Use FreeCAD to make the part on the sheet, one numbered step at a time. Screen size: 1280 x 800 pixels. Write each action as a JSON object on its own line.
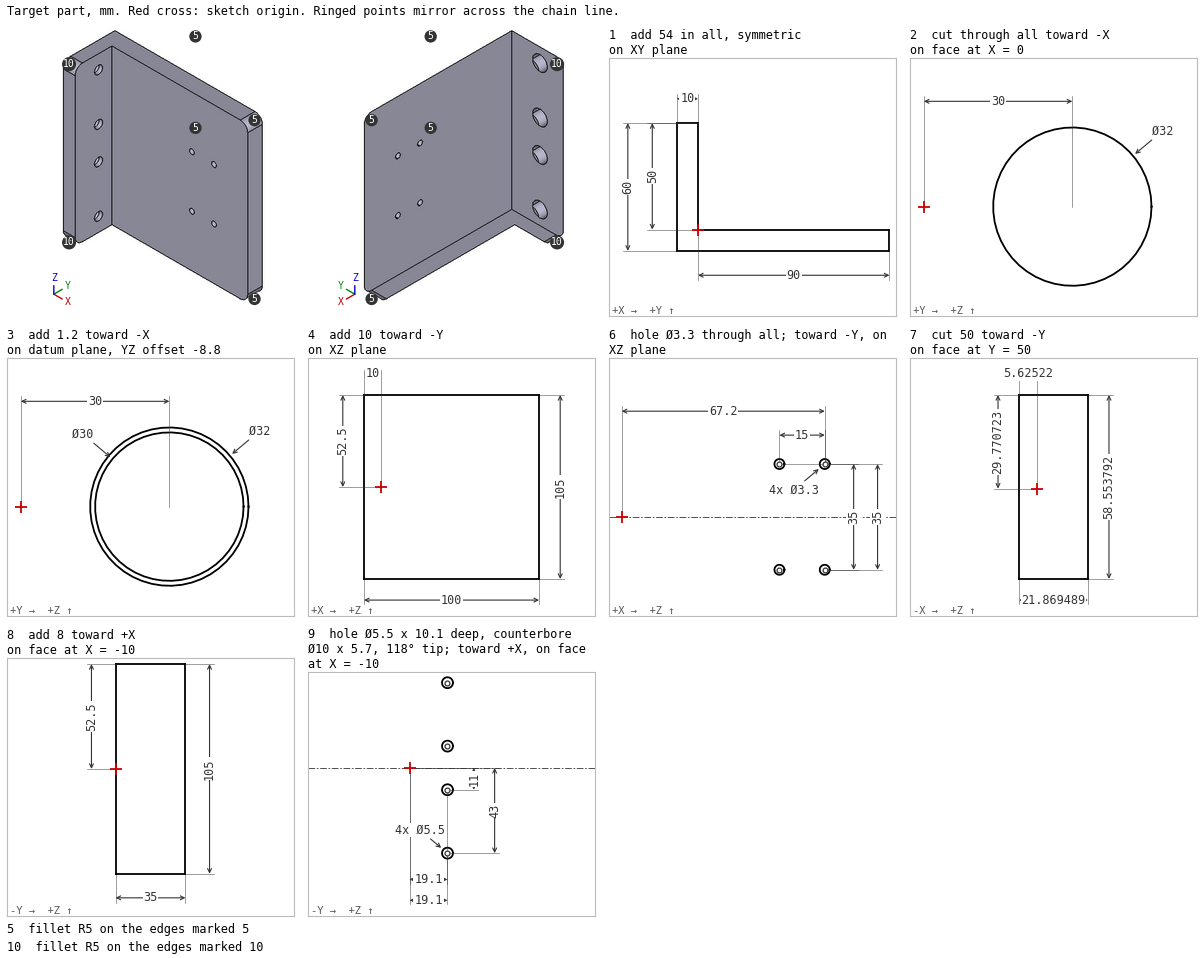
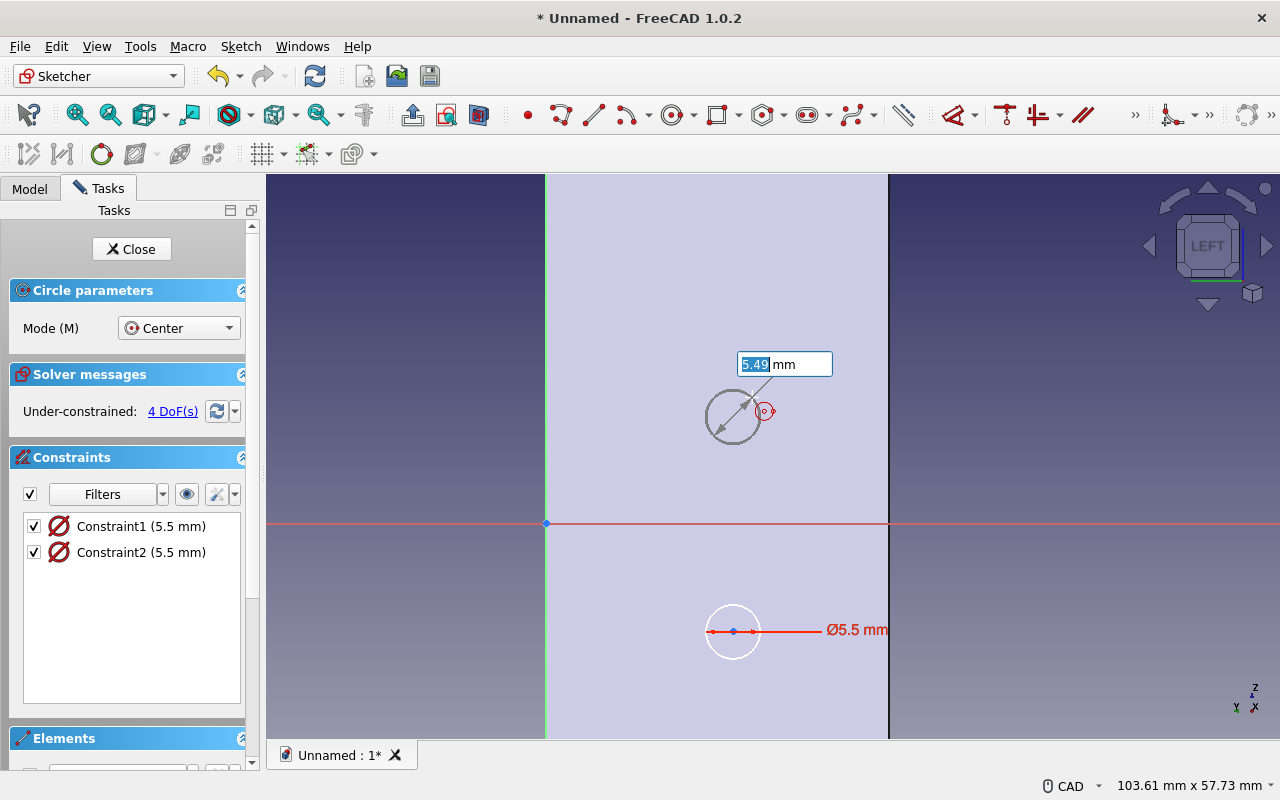
{"action": "type", "text": "5.5"}
{"action": "key", "text": "Return"}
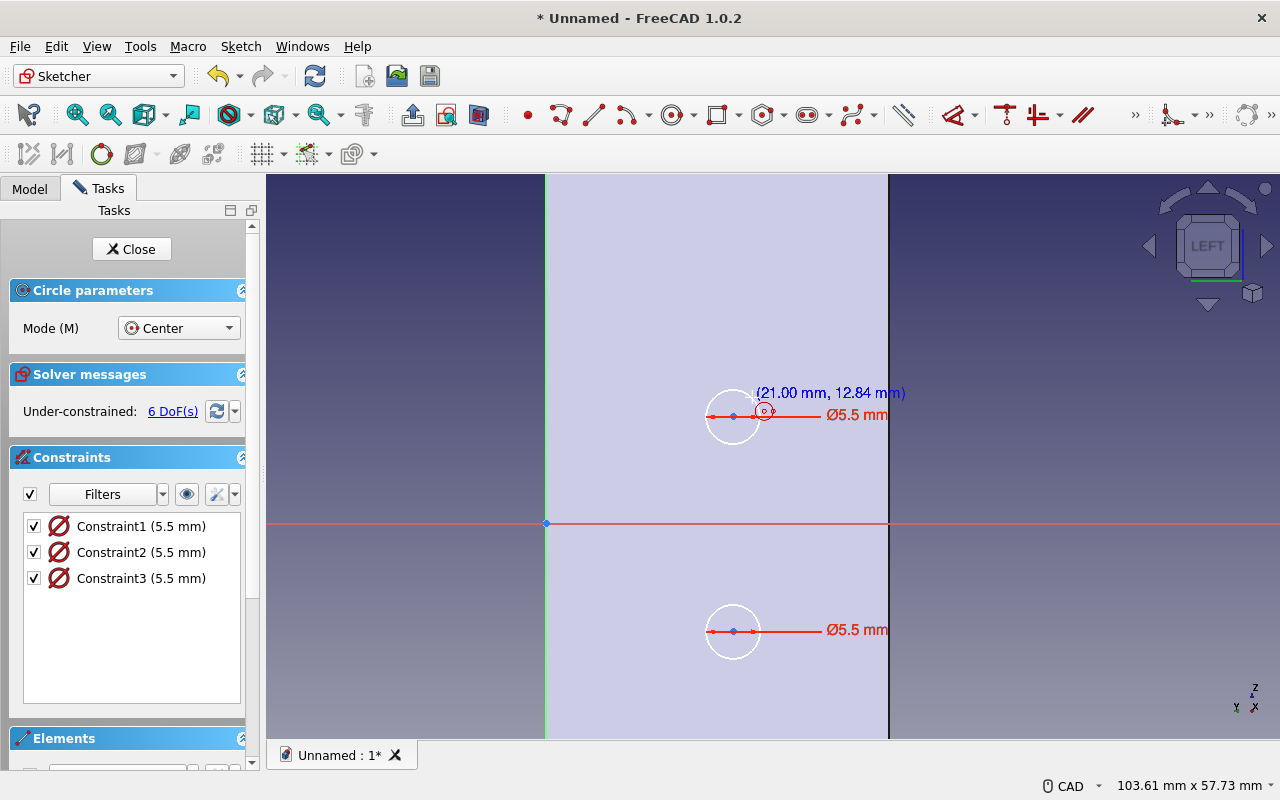
{"action": "scroll", "coordinate": [734, 417], "scroll_direction": "down", "scroll_amount": 5}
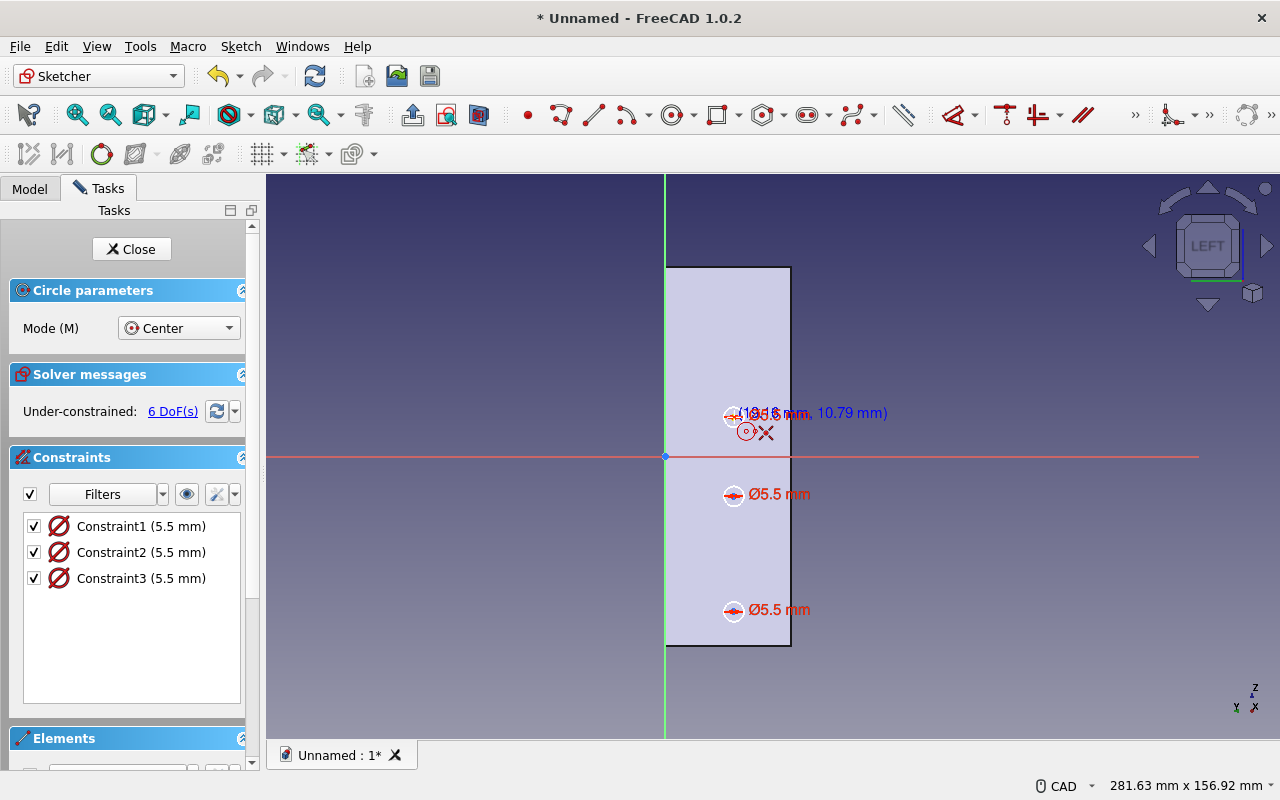
{"action": "scroll", "coordinate": [734, 302], "scroll_direction": "up", "scroll_amount": 5}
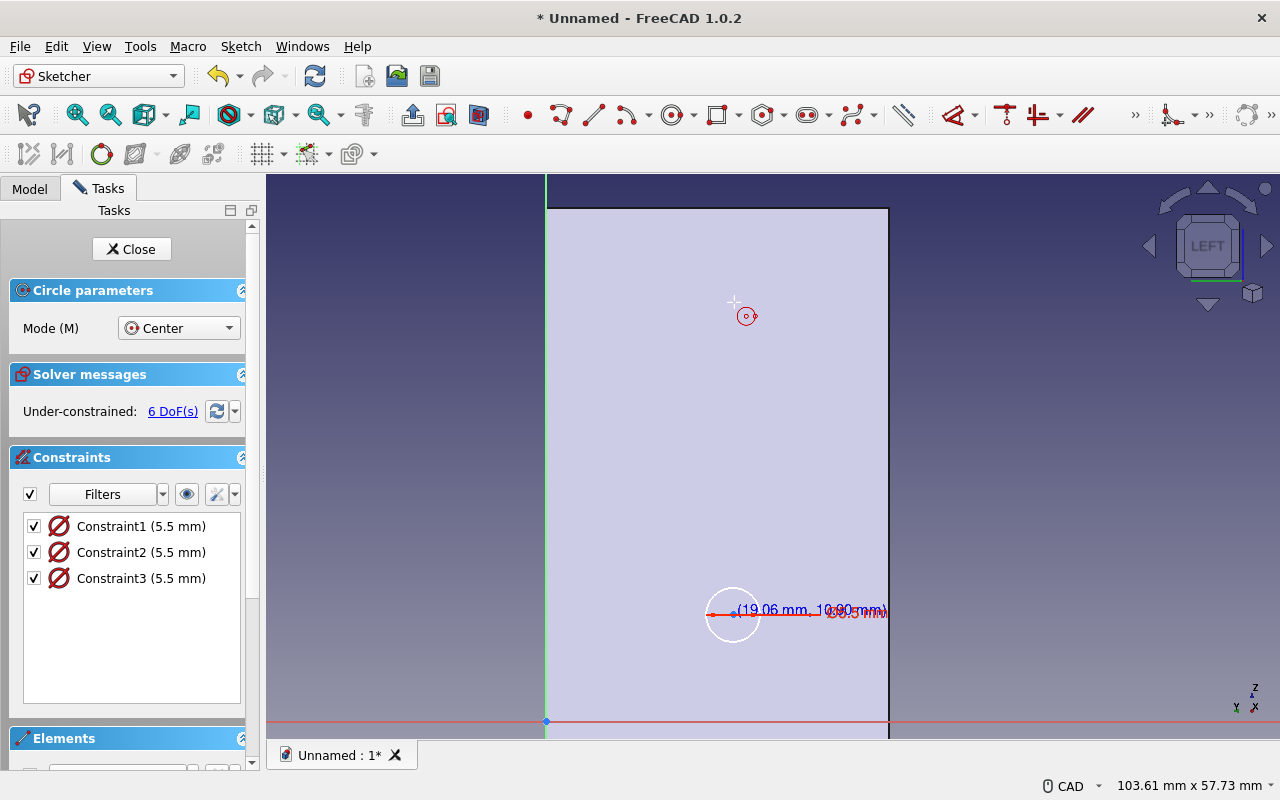
{"action": "left_click", "coordinate": [733, 301]}
{"action": "mouse_move", "coordinate": [752, 282]}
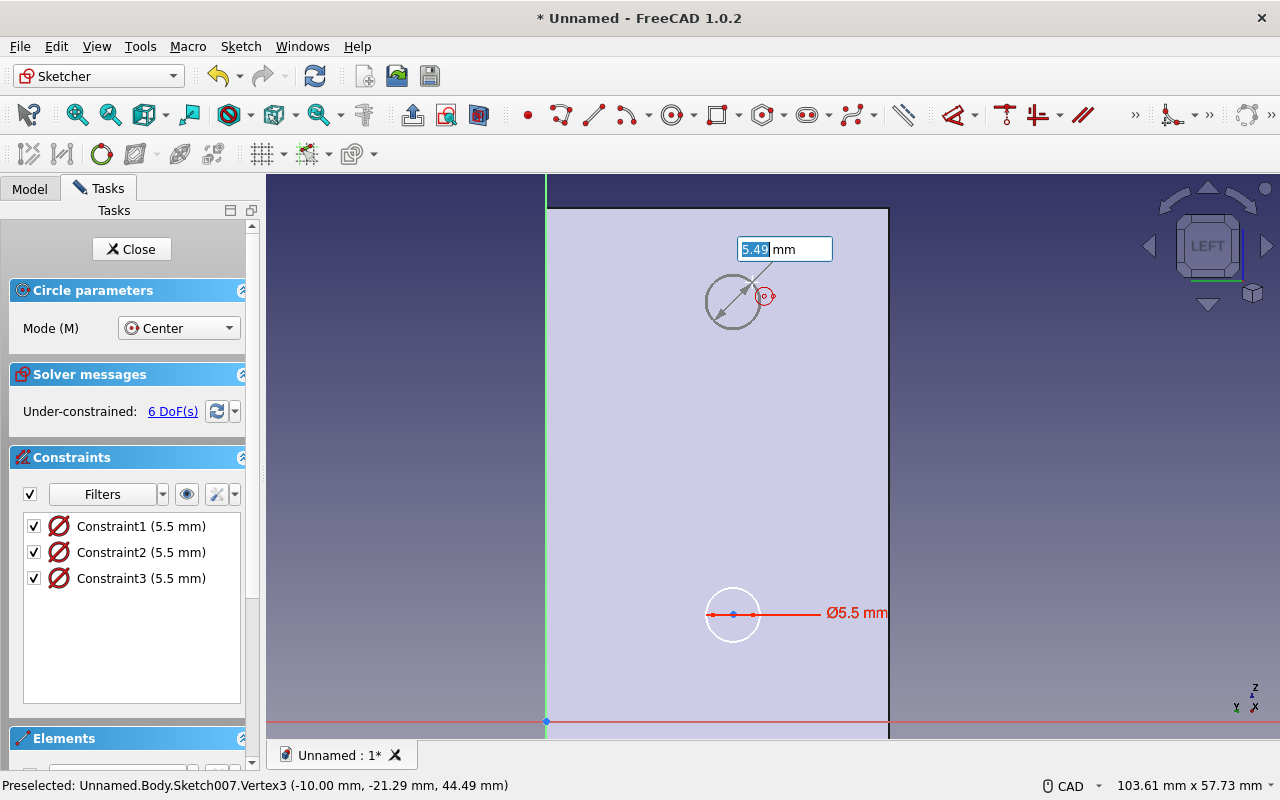
{"action": "type", "text": "5.5"}
{"action": "key", "text": "Return"}
{"action": "key", "text": "Escape"}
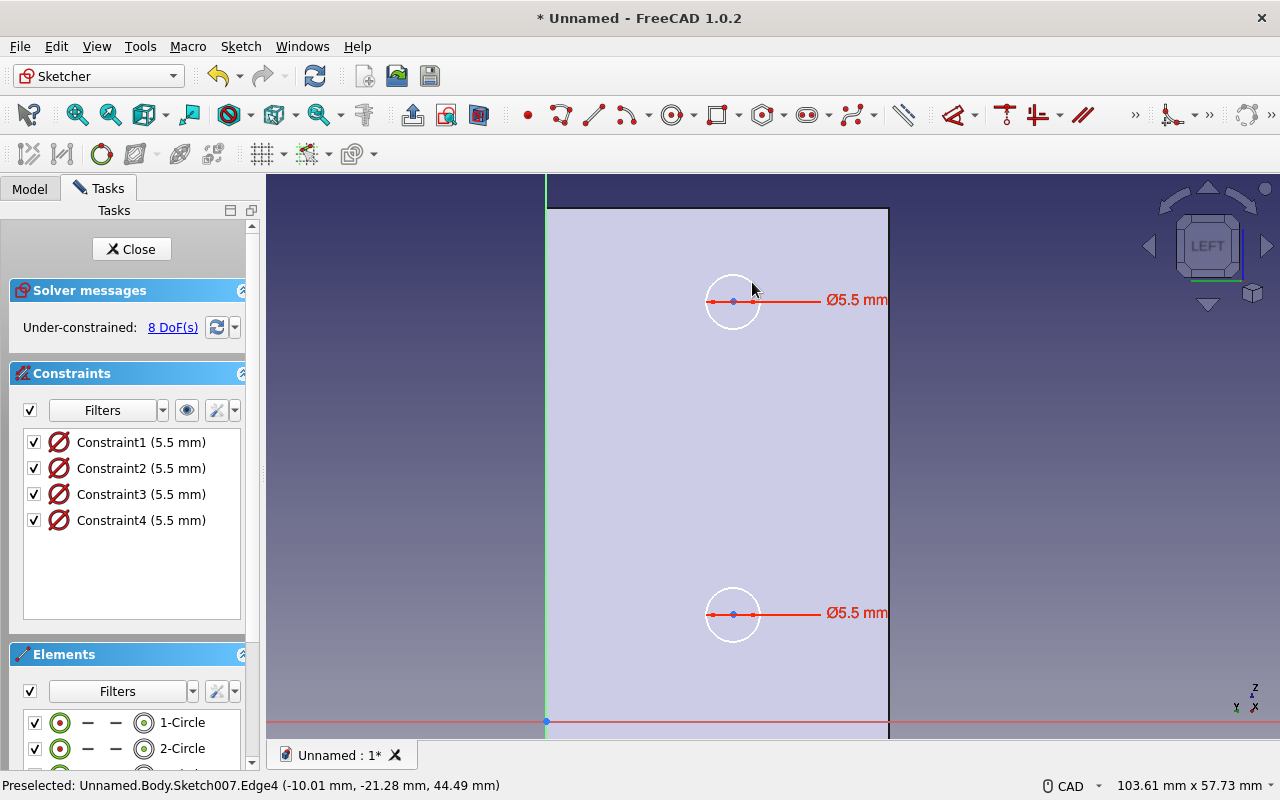
{"action": "scroll", "coordinate": [734, 302], "scroll_direction": "down", "scroll_amount": 5}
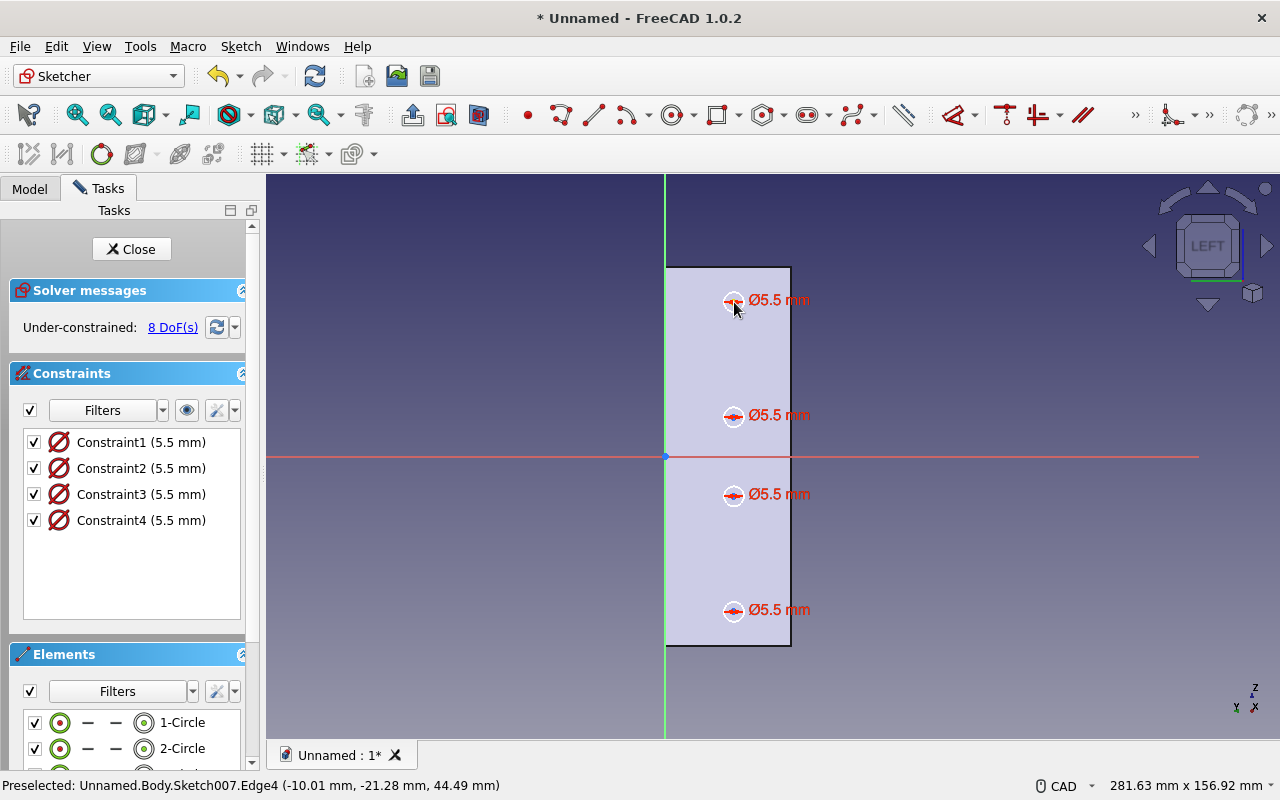
{"action": "left_click", "coordinate": [734, 496]}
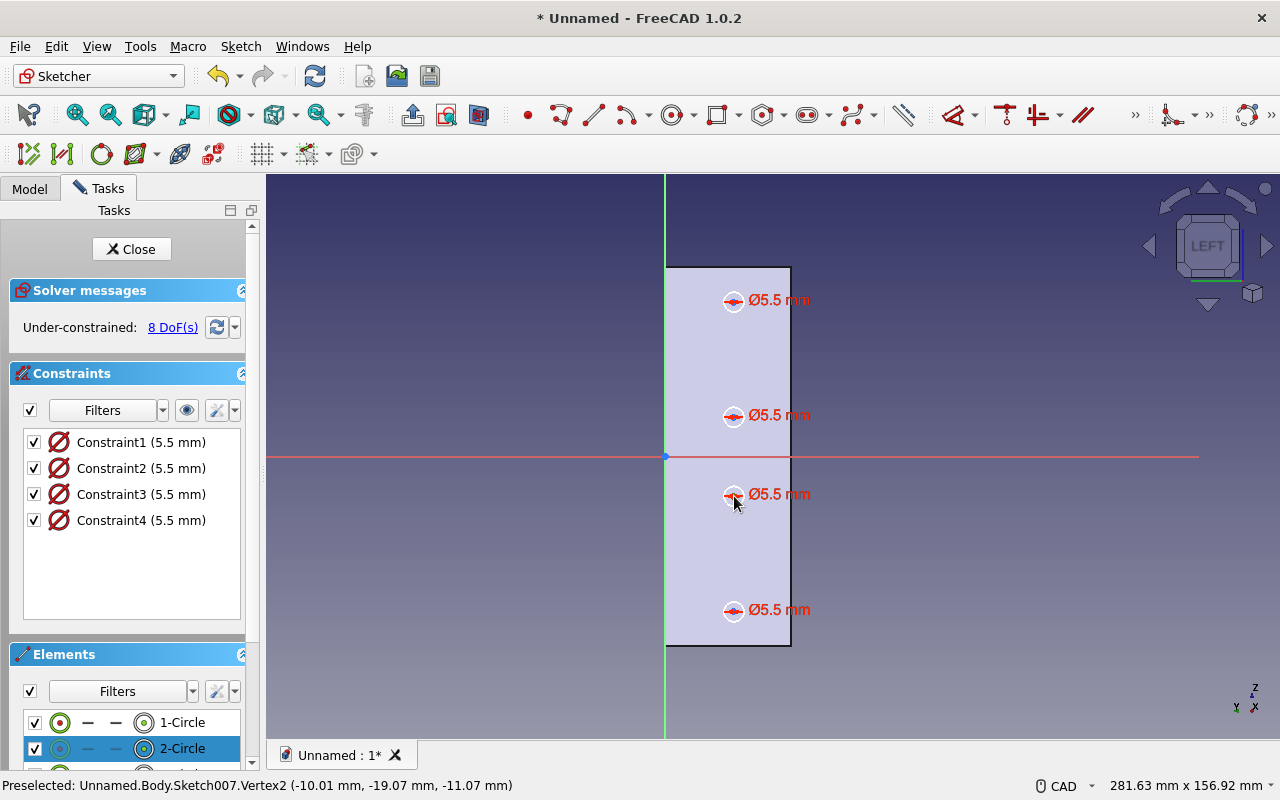
{"action": "left_click", "coordinate": [734, 417]}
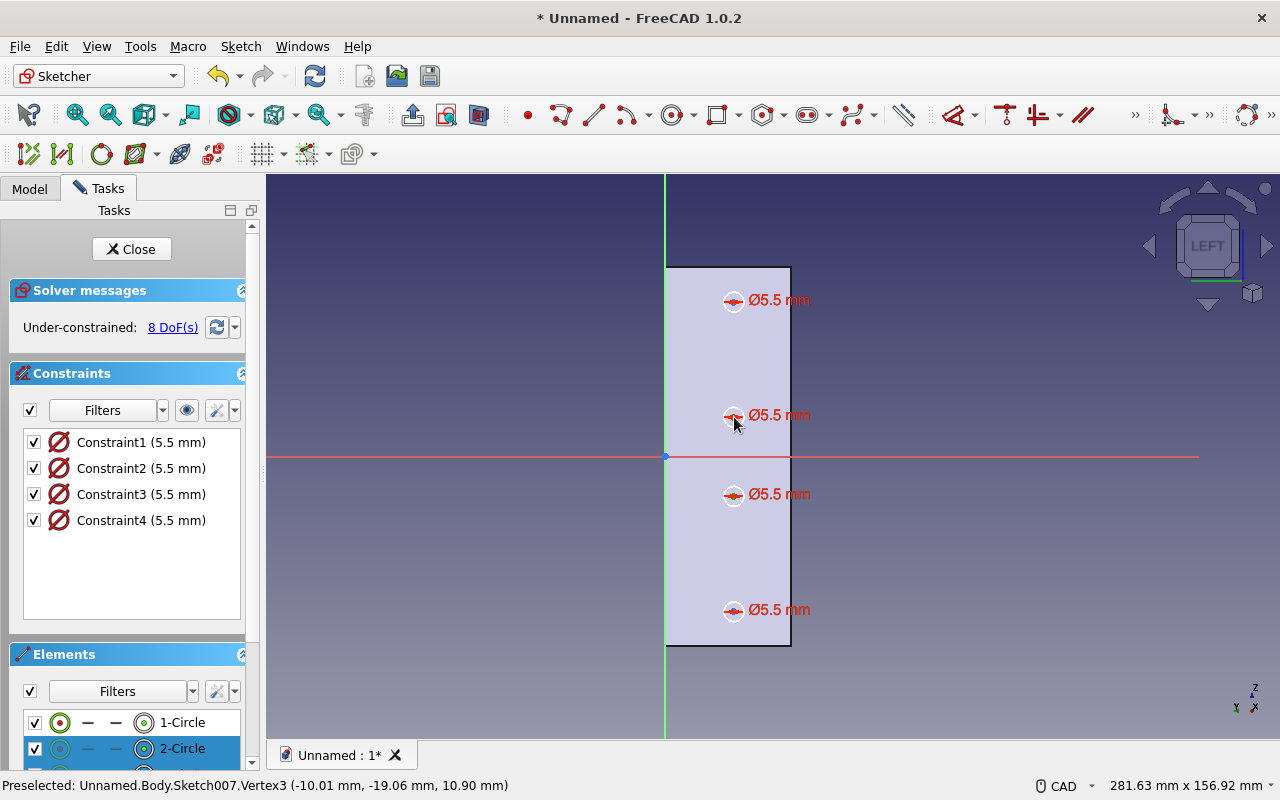
{"action": "left_click", "coordinate": [353, 457]}